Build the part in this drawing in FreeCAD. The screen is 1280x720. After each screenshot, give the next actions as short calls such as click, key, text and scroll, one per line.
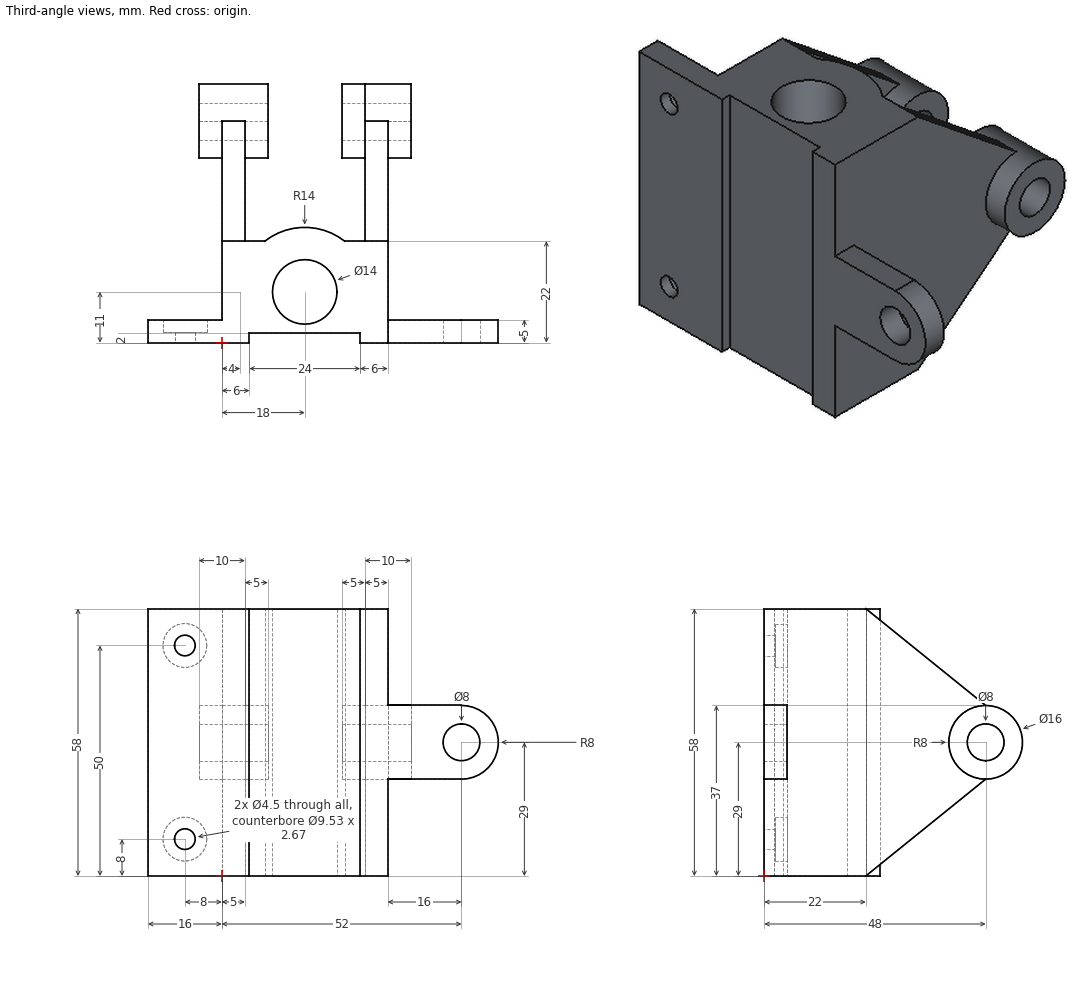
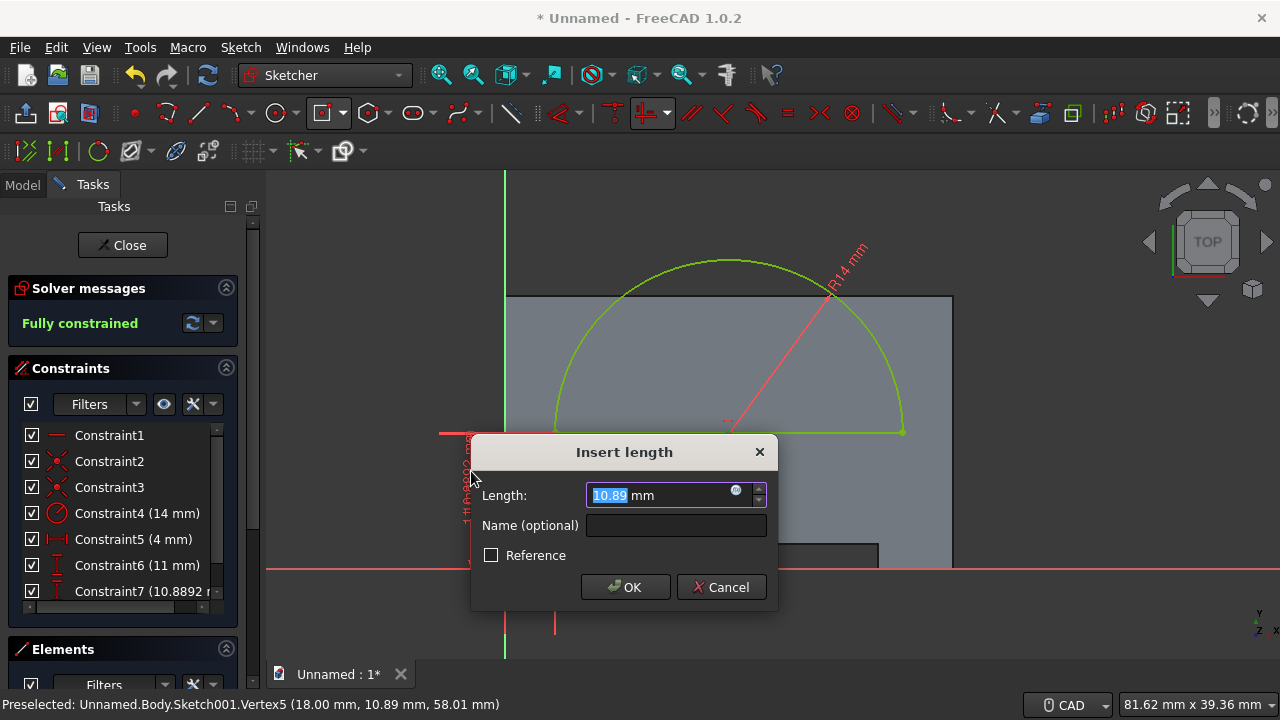
text(11)
key(Return)
key(Escape)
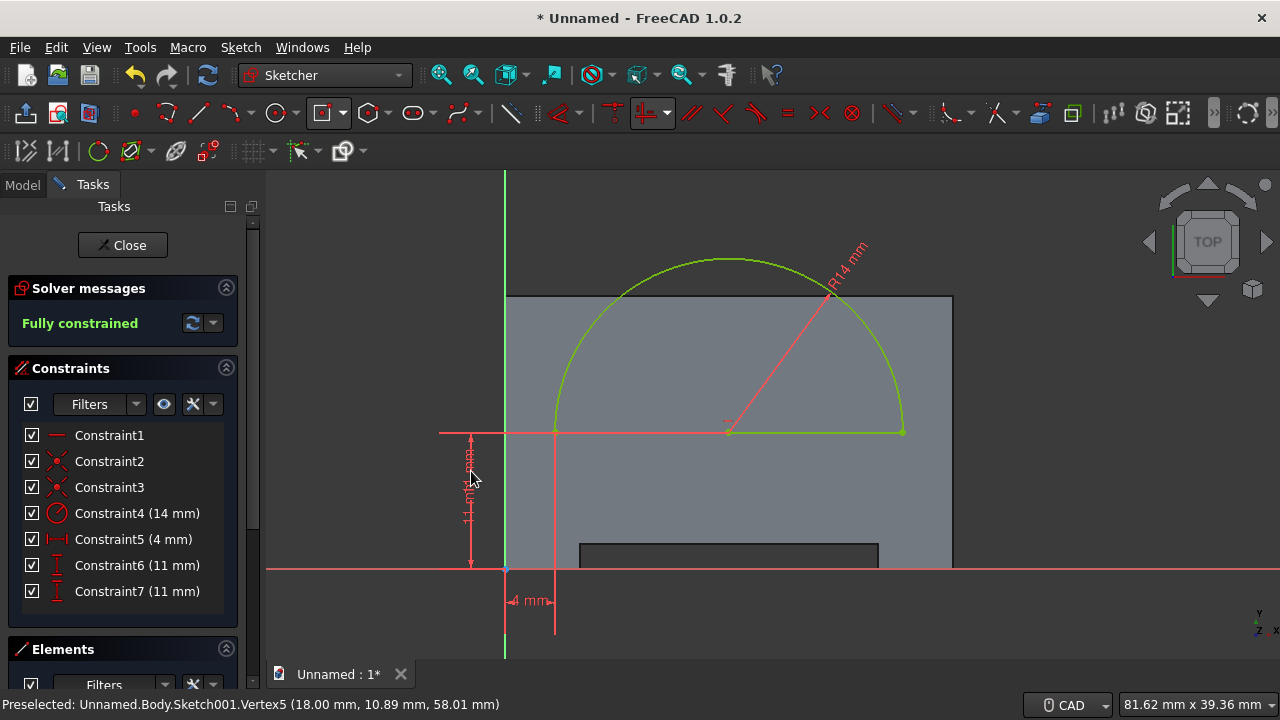
click(123, 245)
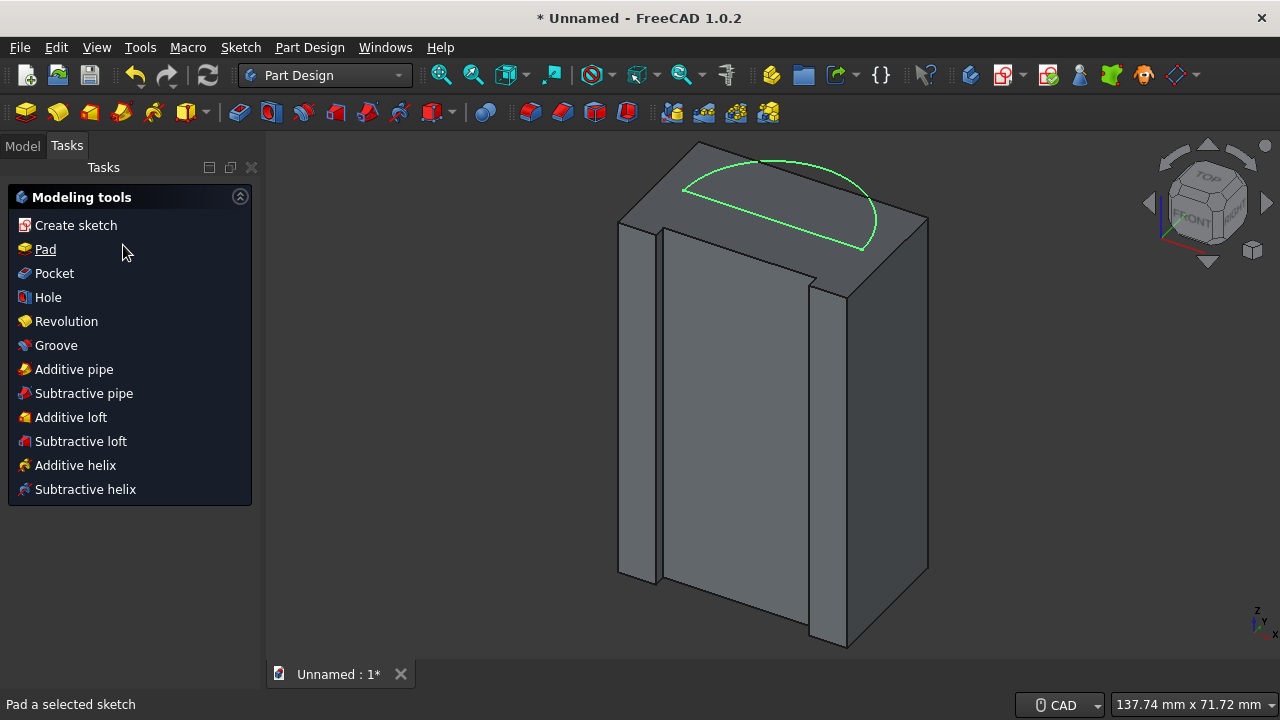
click(26, 112)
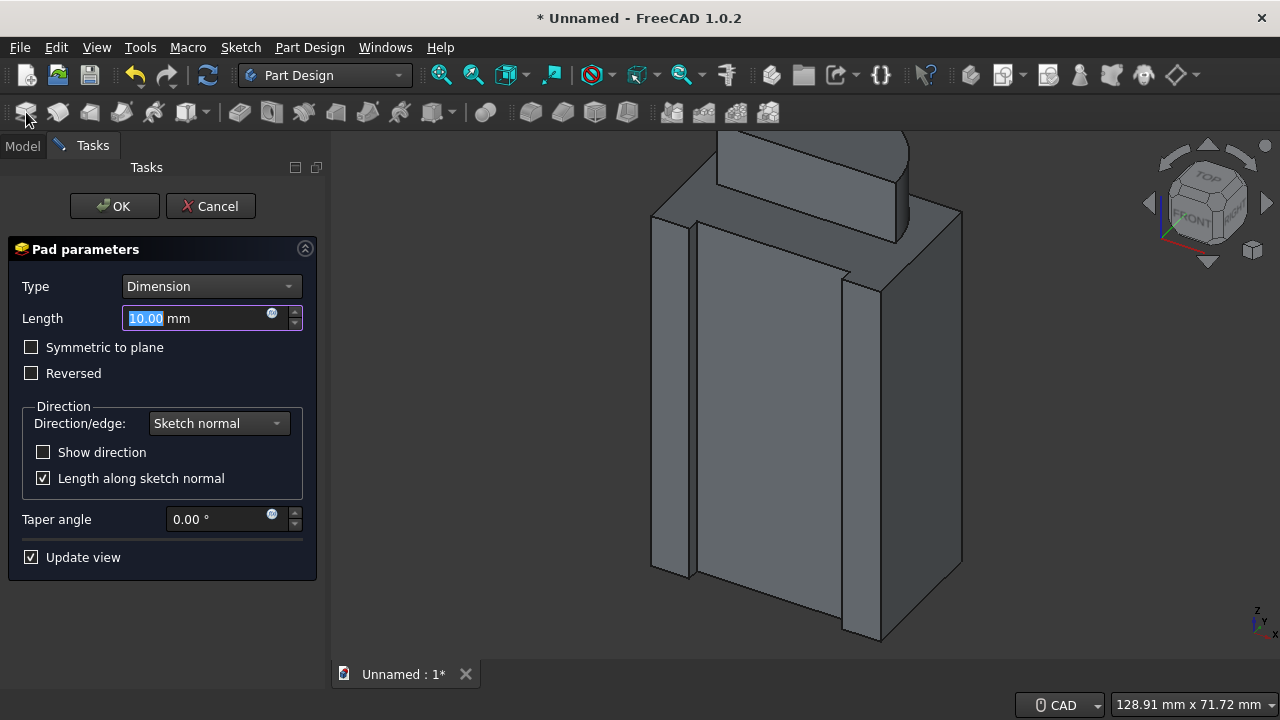
text(58)
key(Tab)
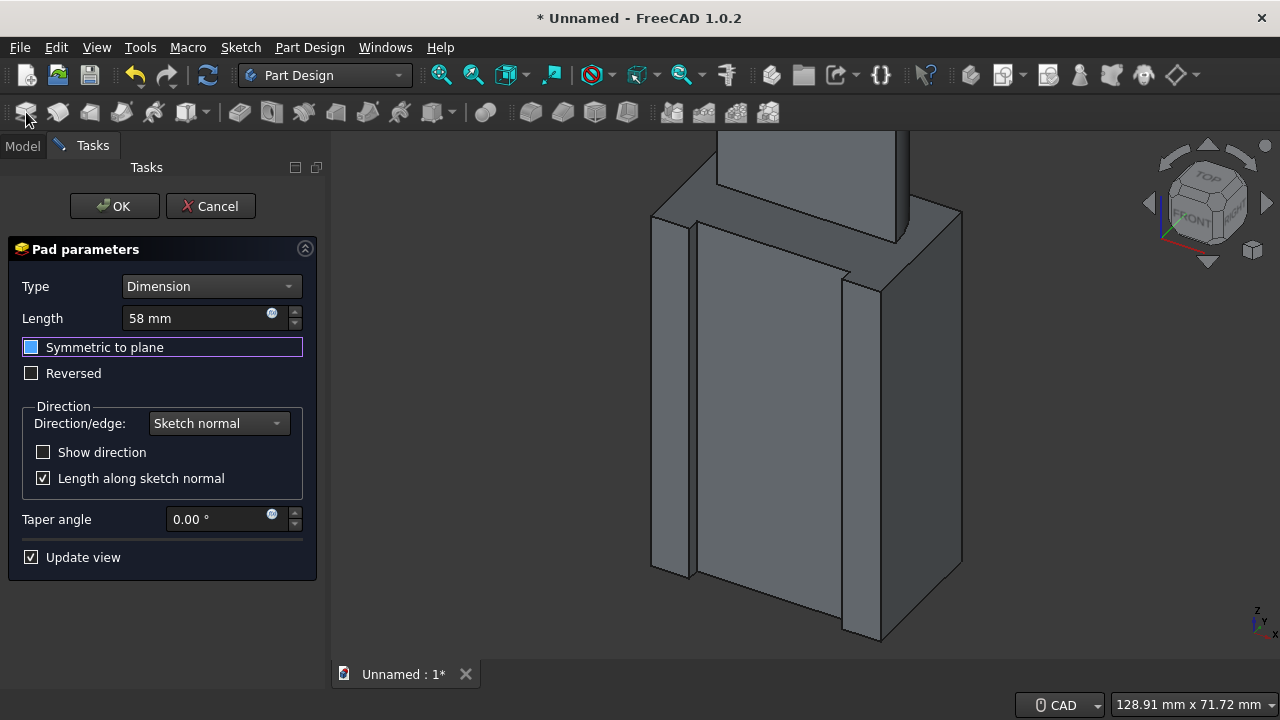
click(30, 373)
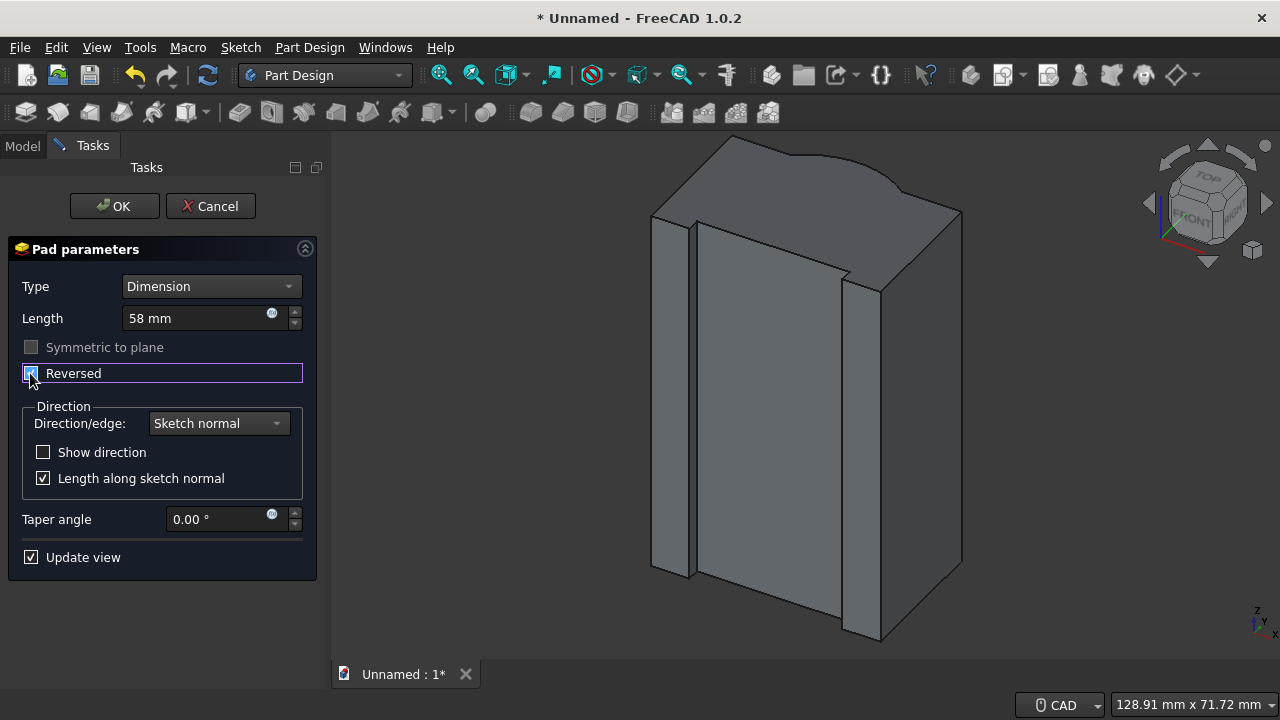
click(115, 206)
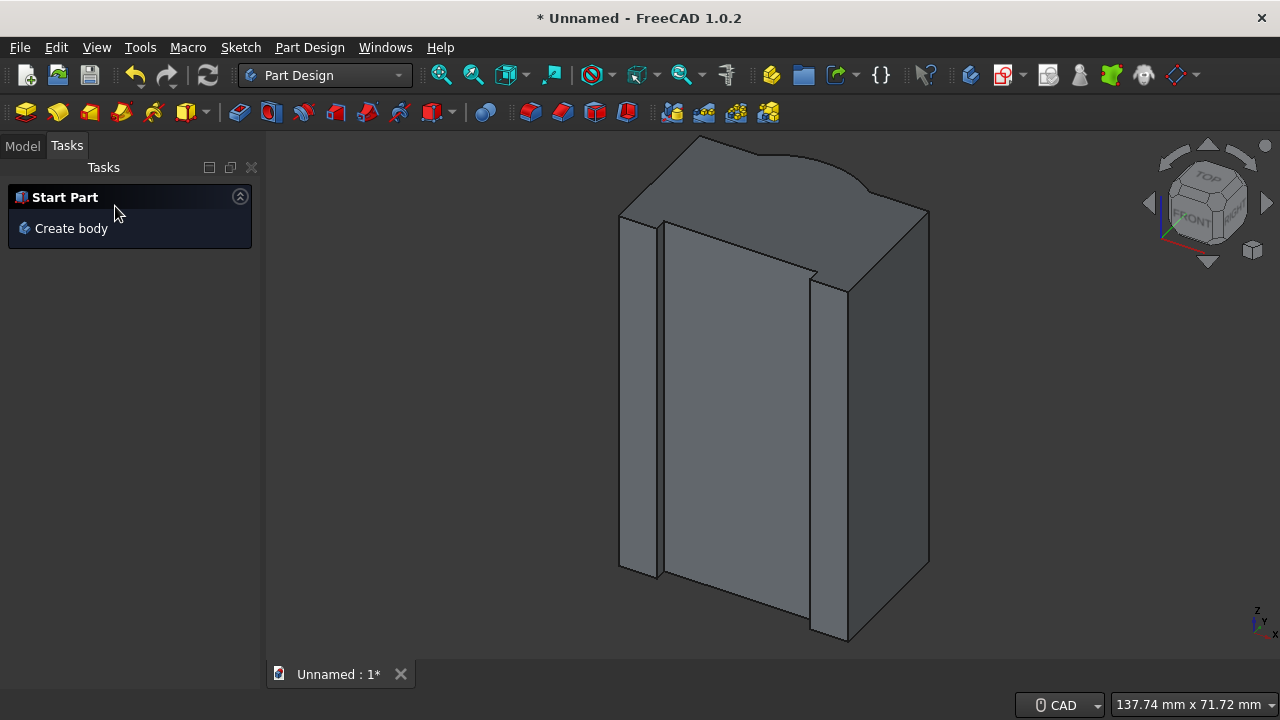
key(v)
key(f)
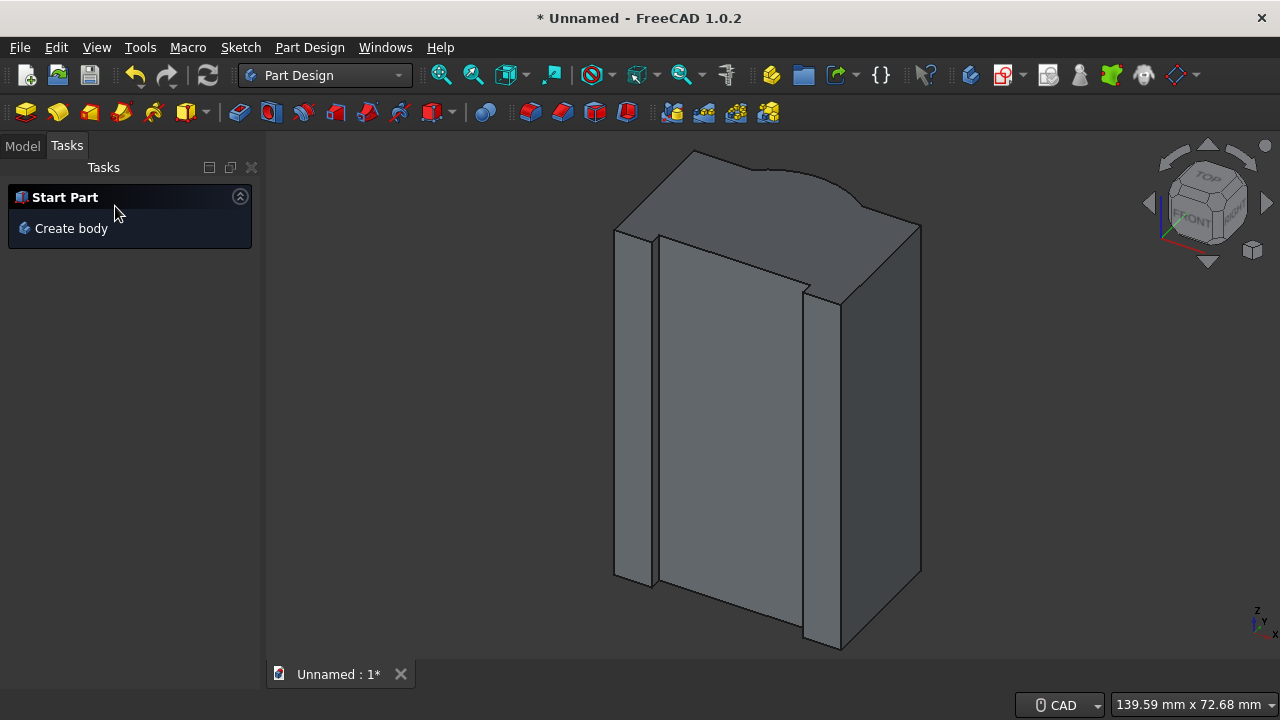
click(773, 221)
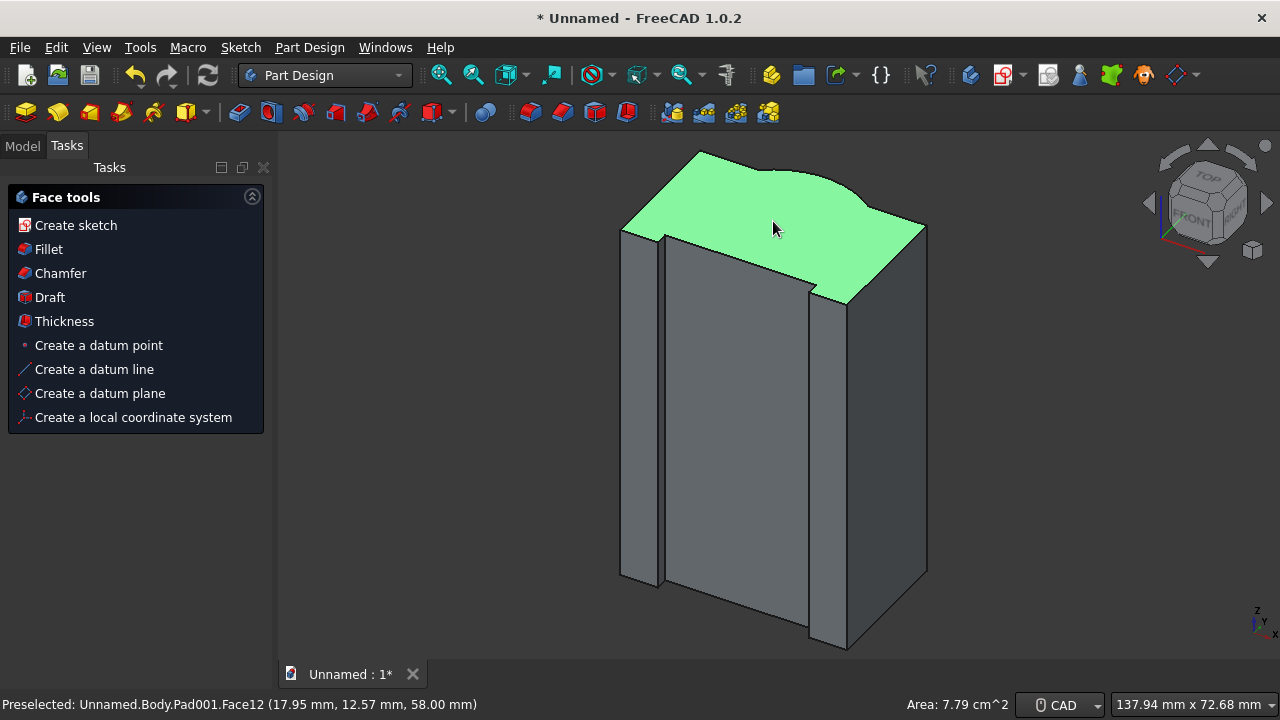
click(1004, 76)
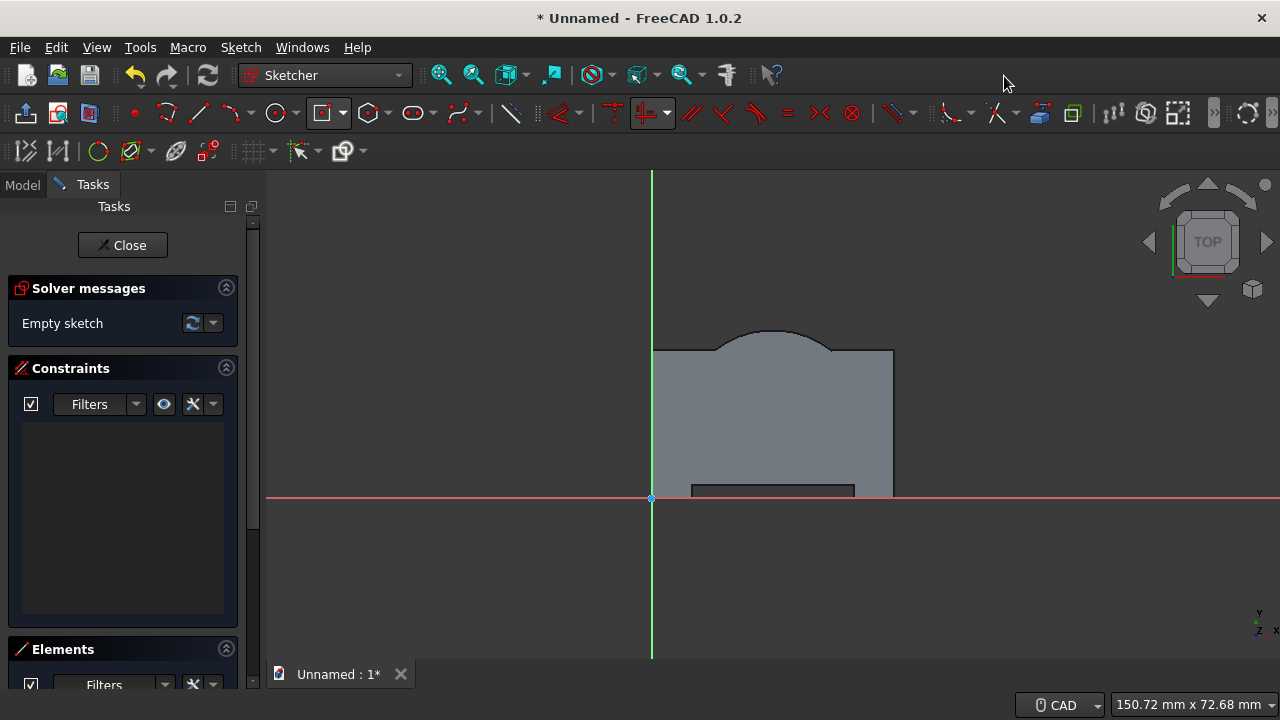
scroll(754, 452, up, 5)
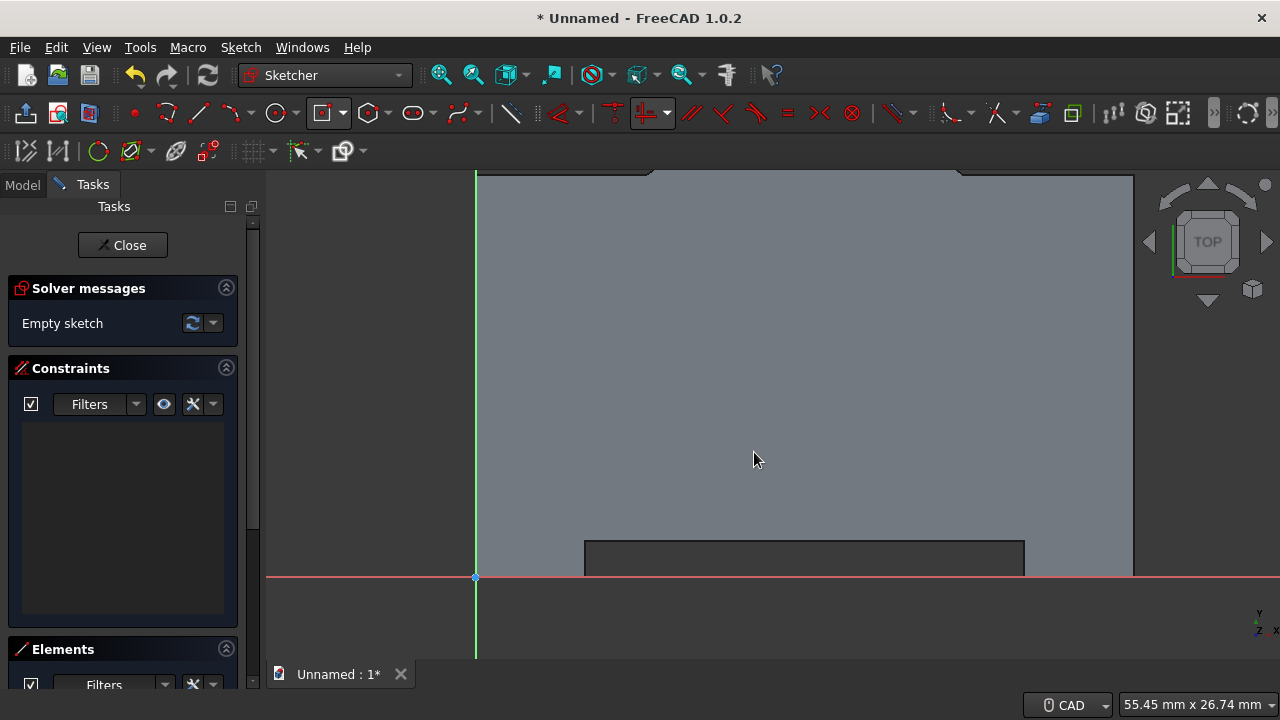
click(276, 114)